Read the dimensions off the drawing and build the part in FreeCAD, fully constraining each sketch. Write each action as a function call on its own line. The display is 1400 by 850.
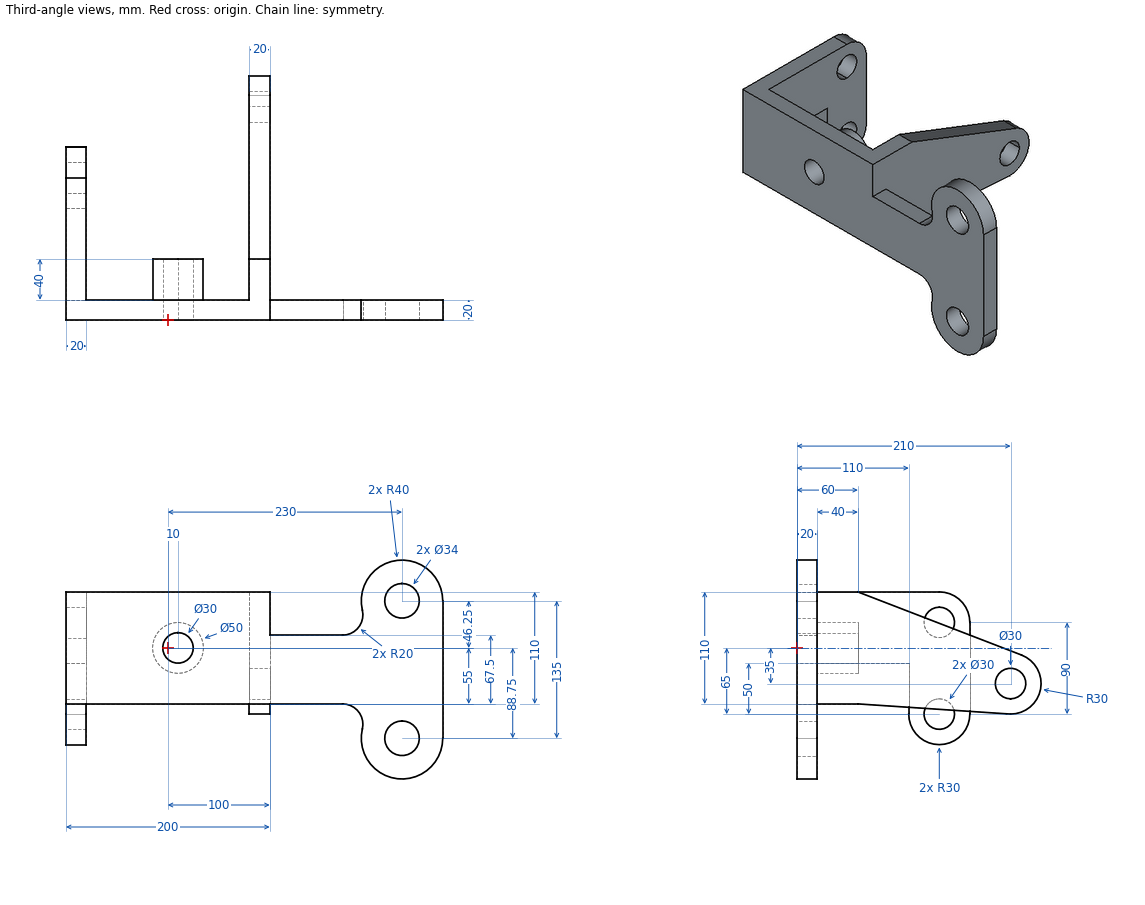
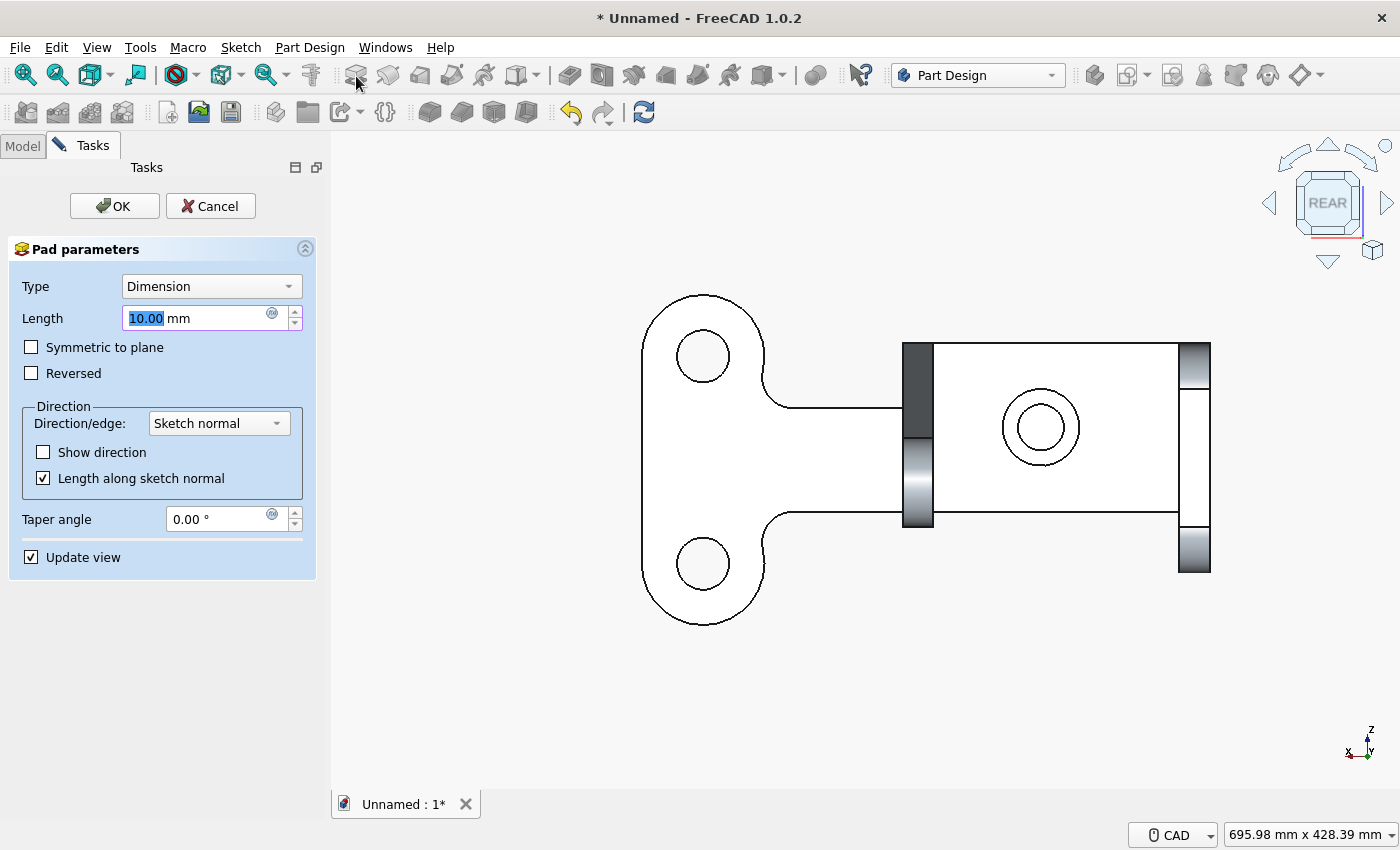
text(40)
key(Tab)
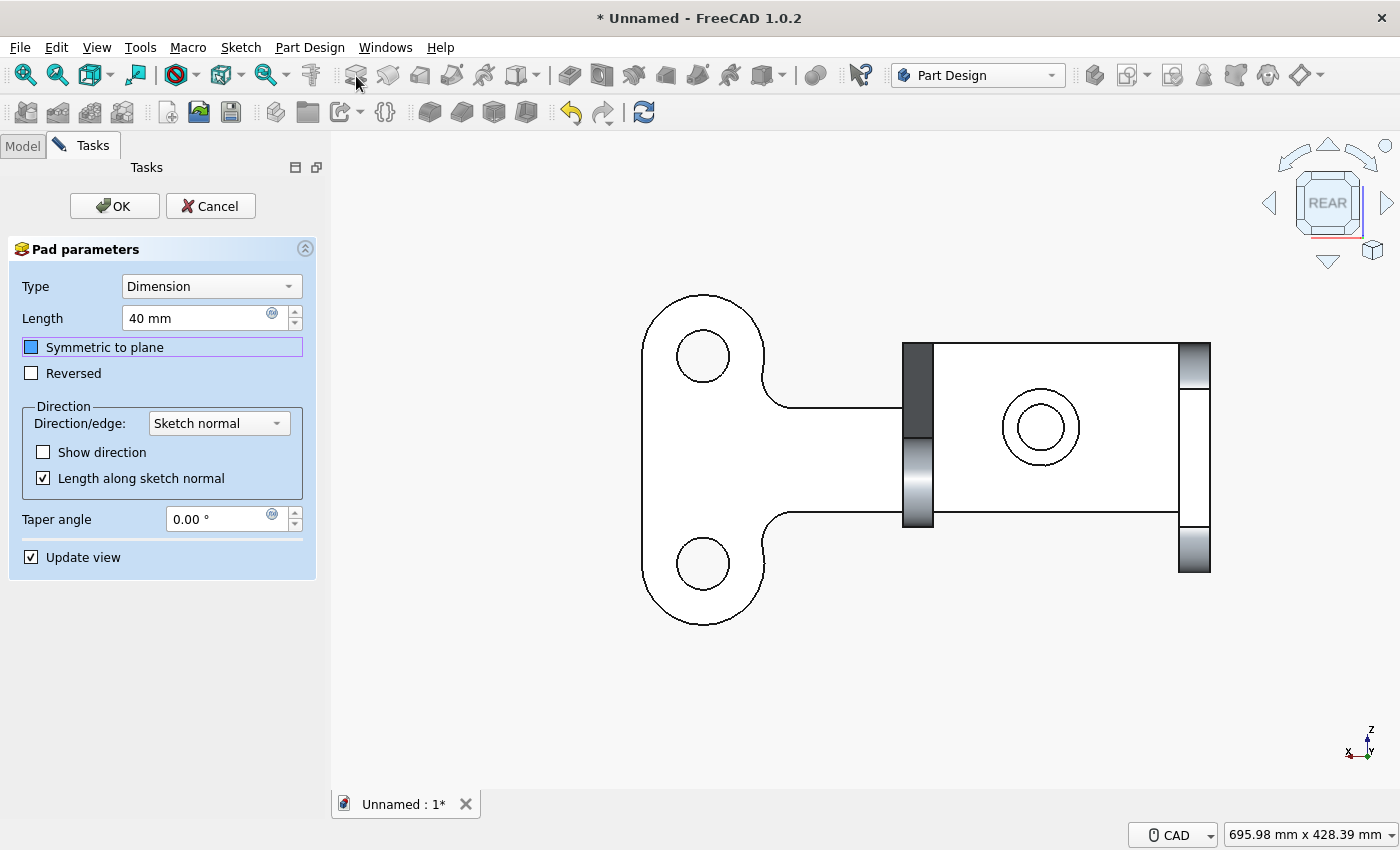
click(115, 206)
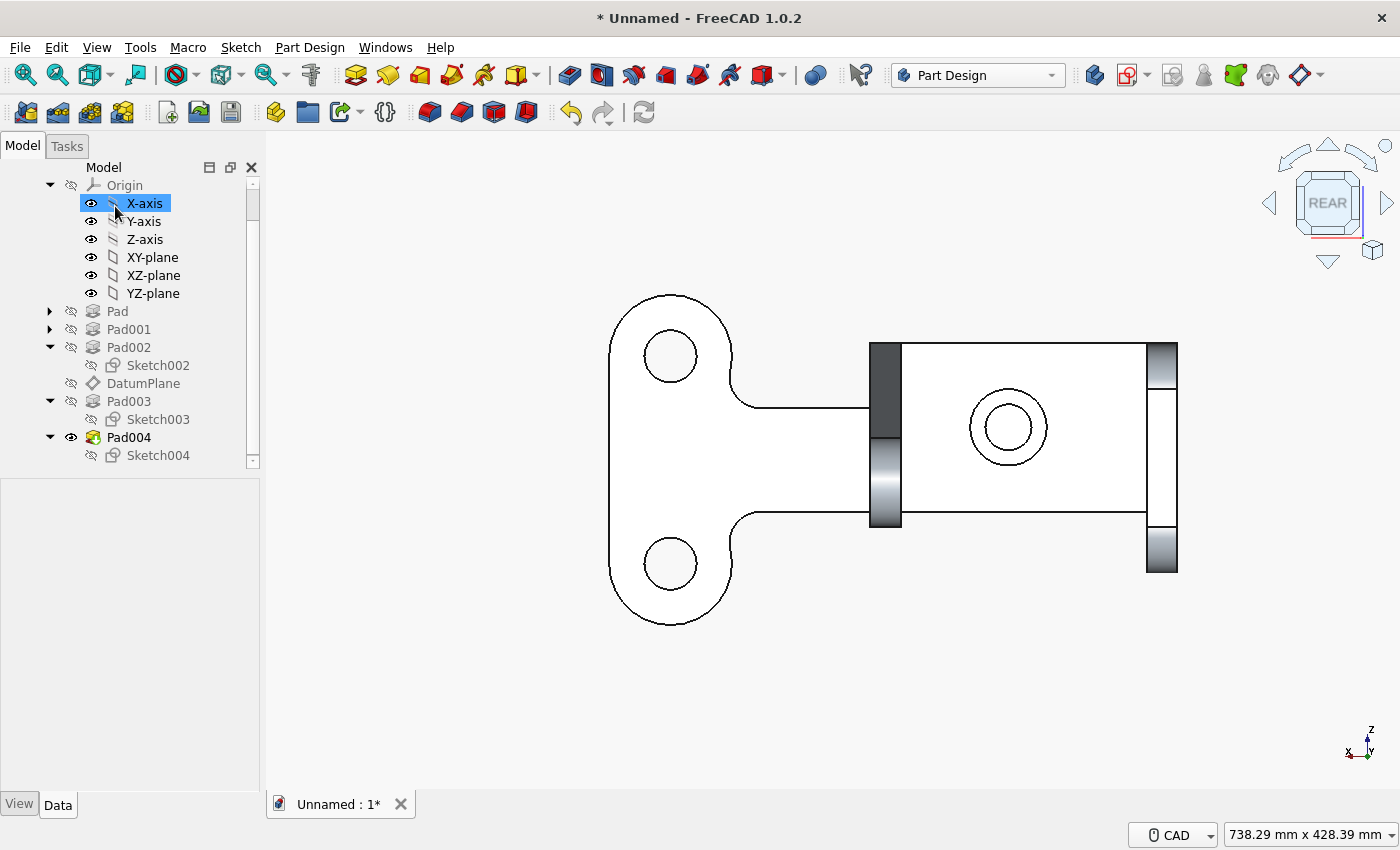
click(136, 275)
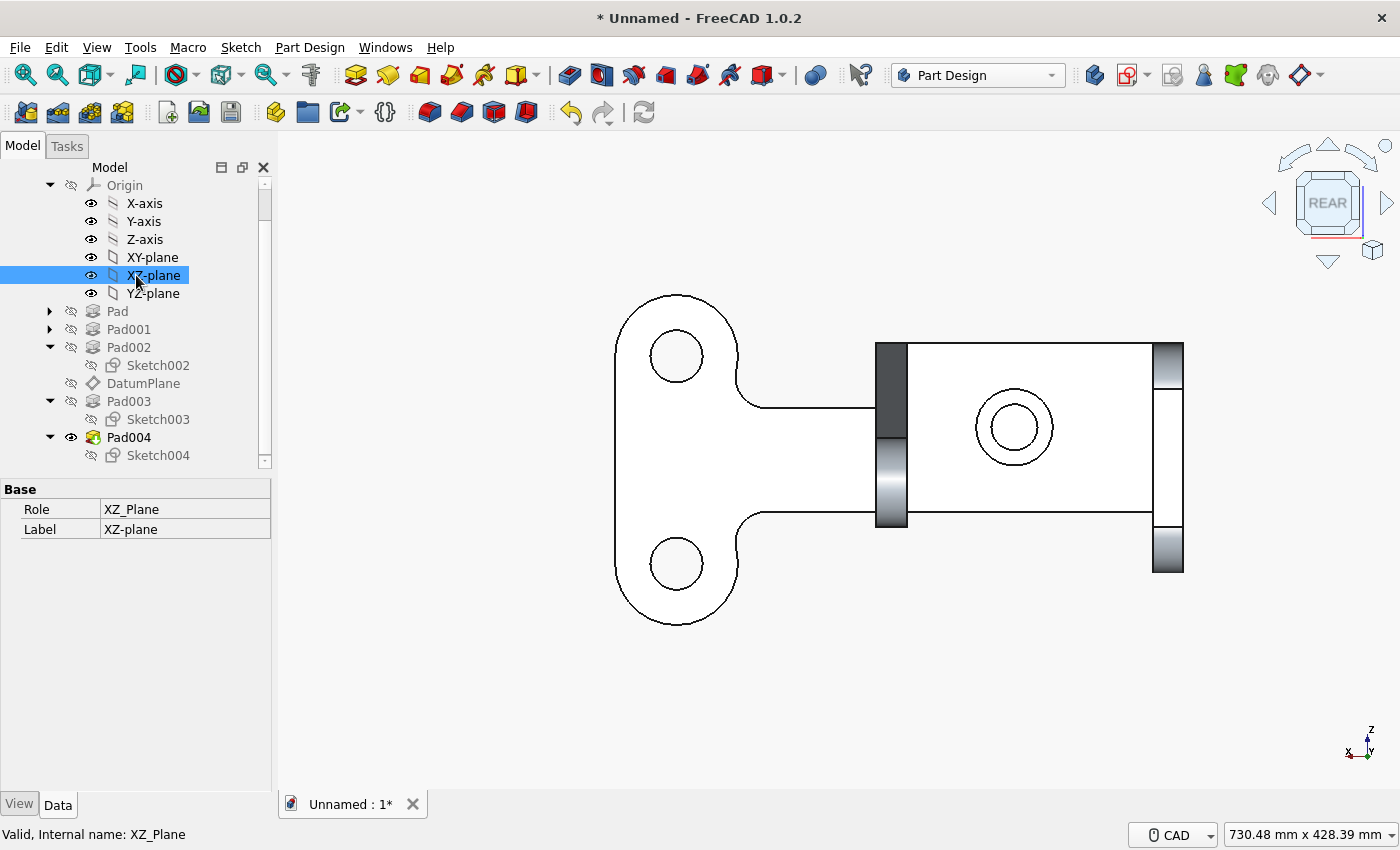
click(1300, 76)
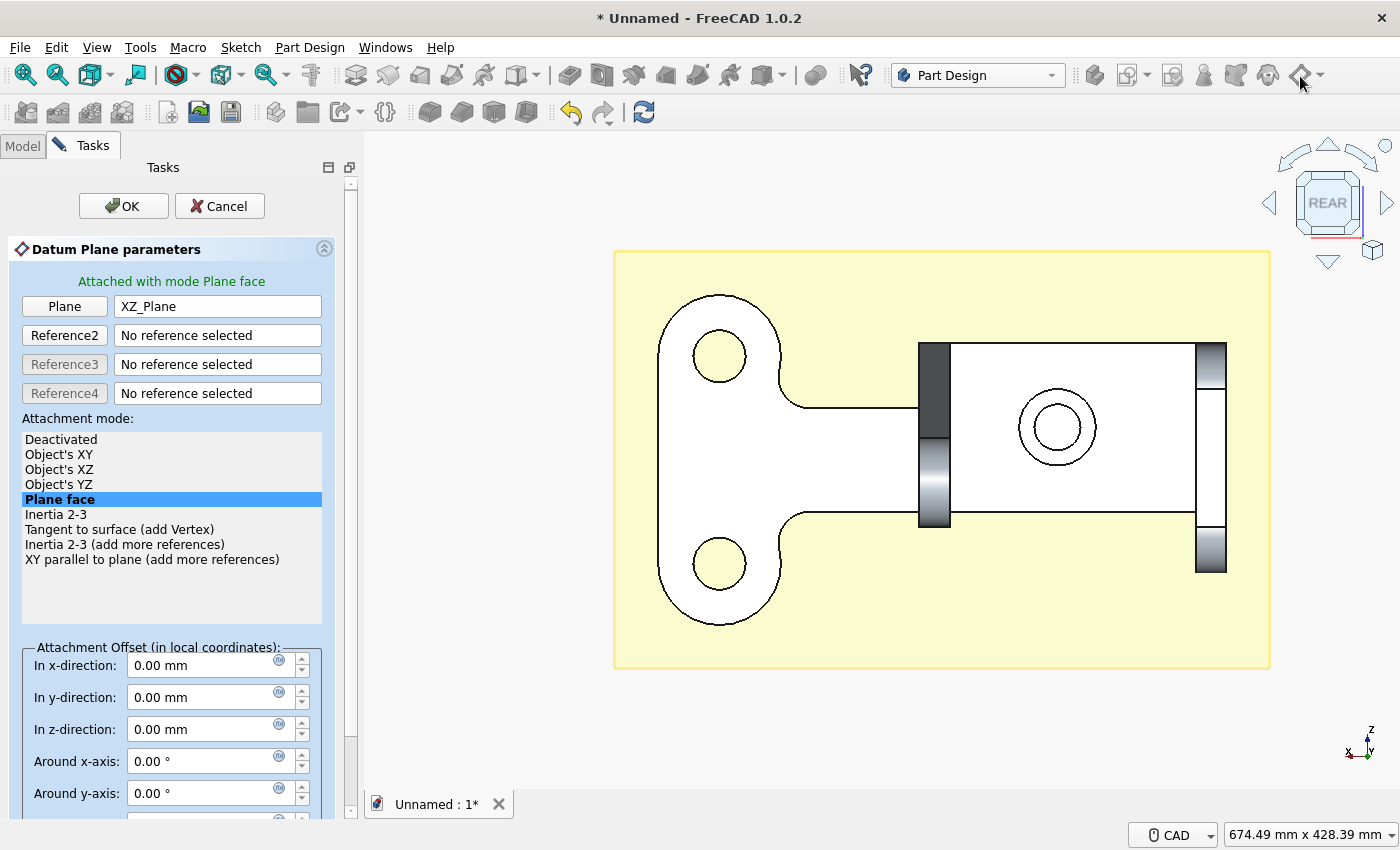
triple_click(210, 729)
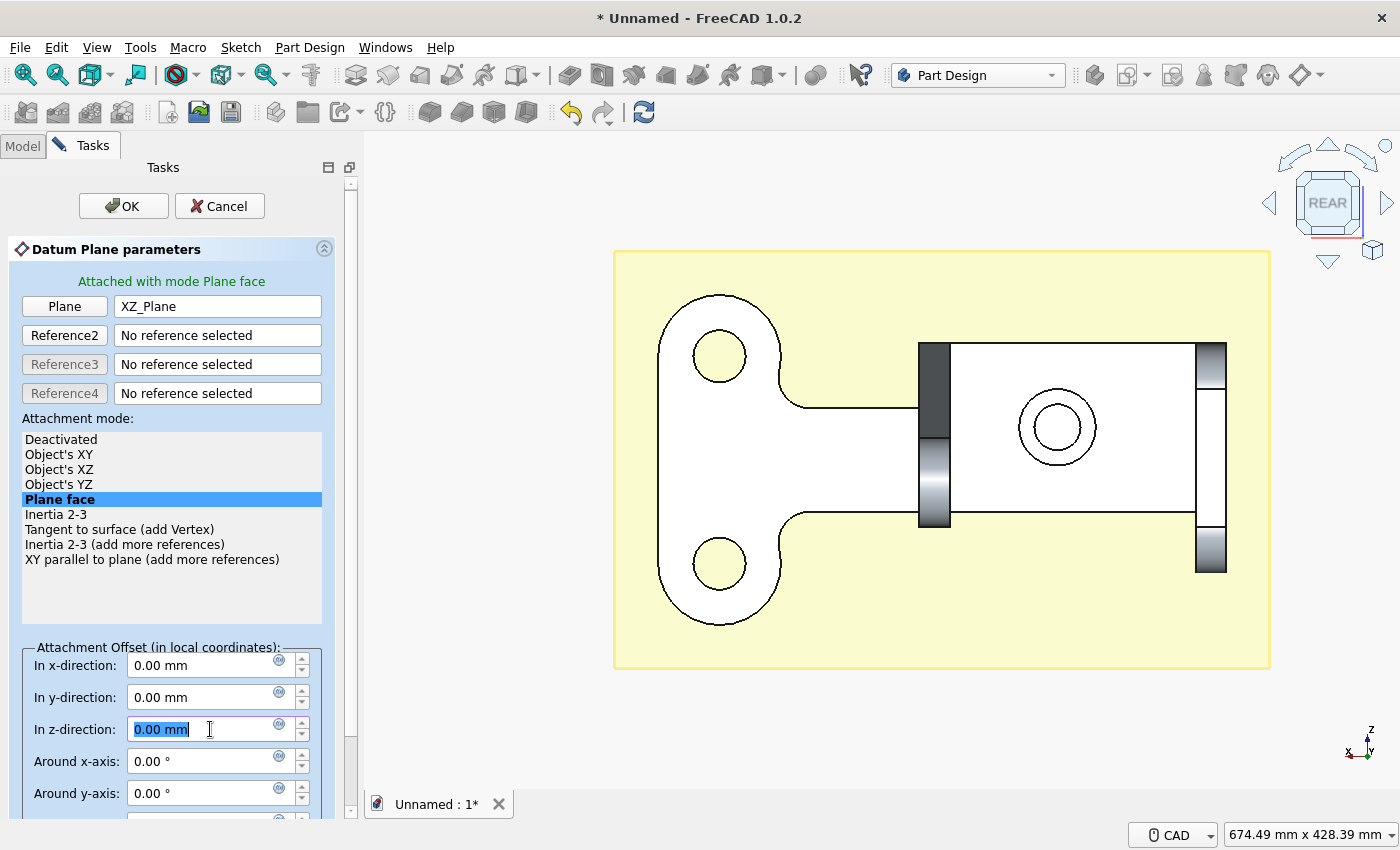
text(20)
key(Tab)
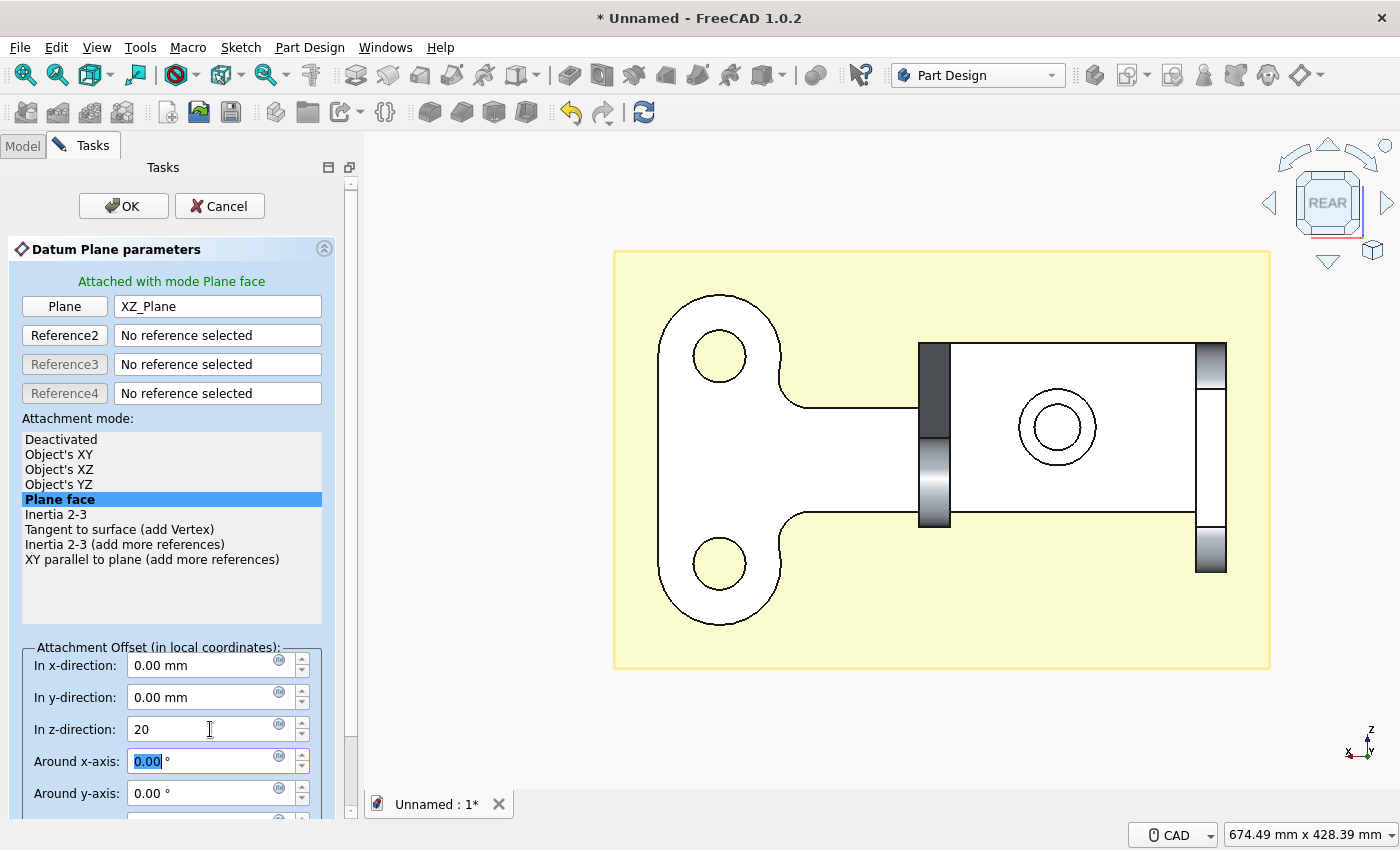
click(124, 206)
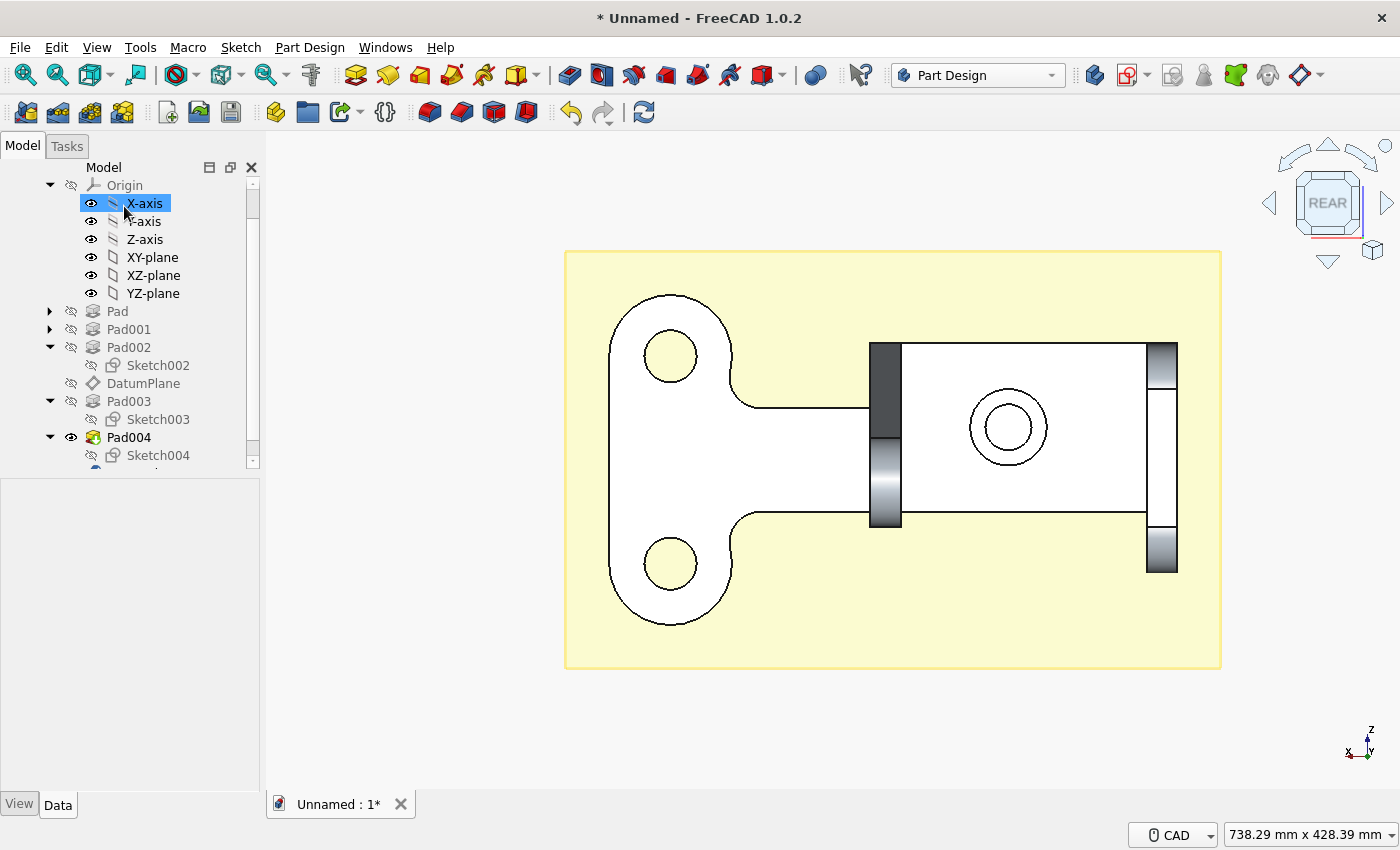
scroll(140, 325, down, 3)